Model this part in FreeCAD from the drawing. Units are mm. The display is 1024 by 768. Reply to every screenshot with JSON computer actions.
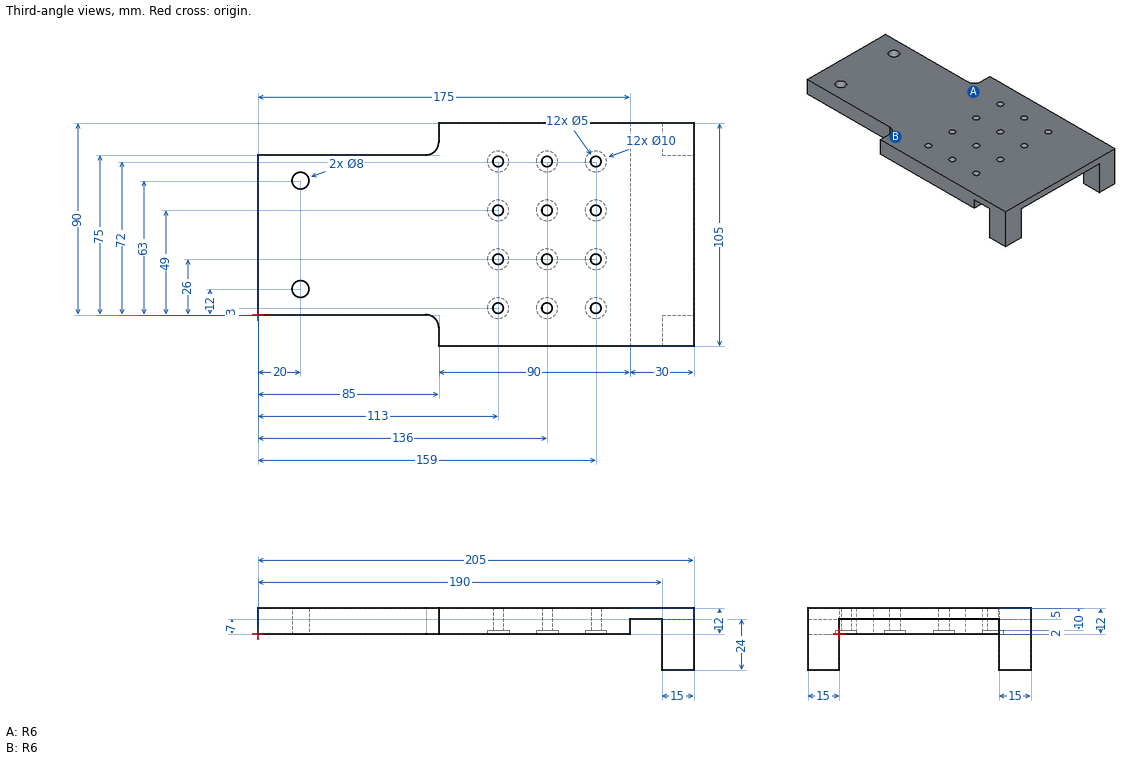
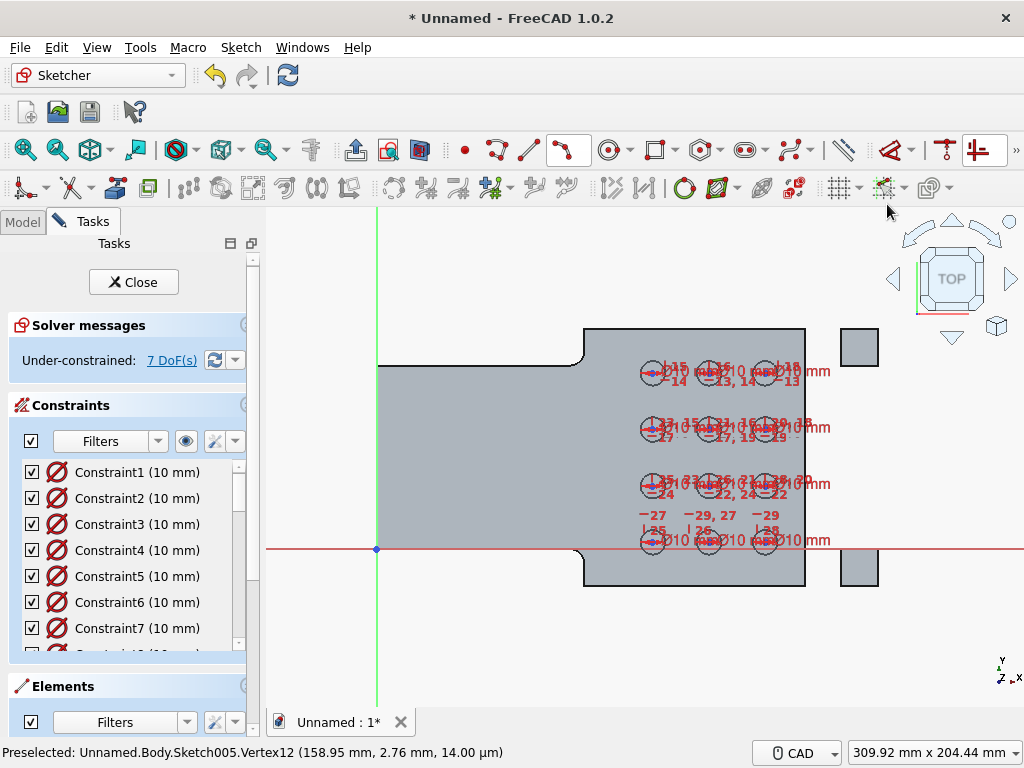
{"action": "key", "text": "d"}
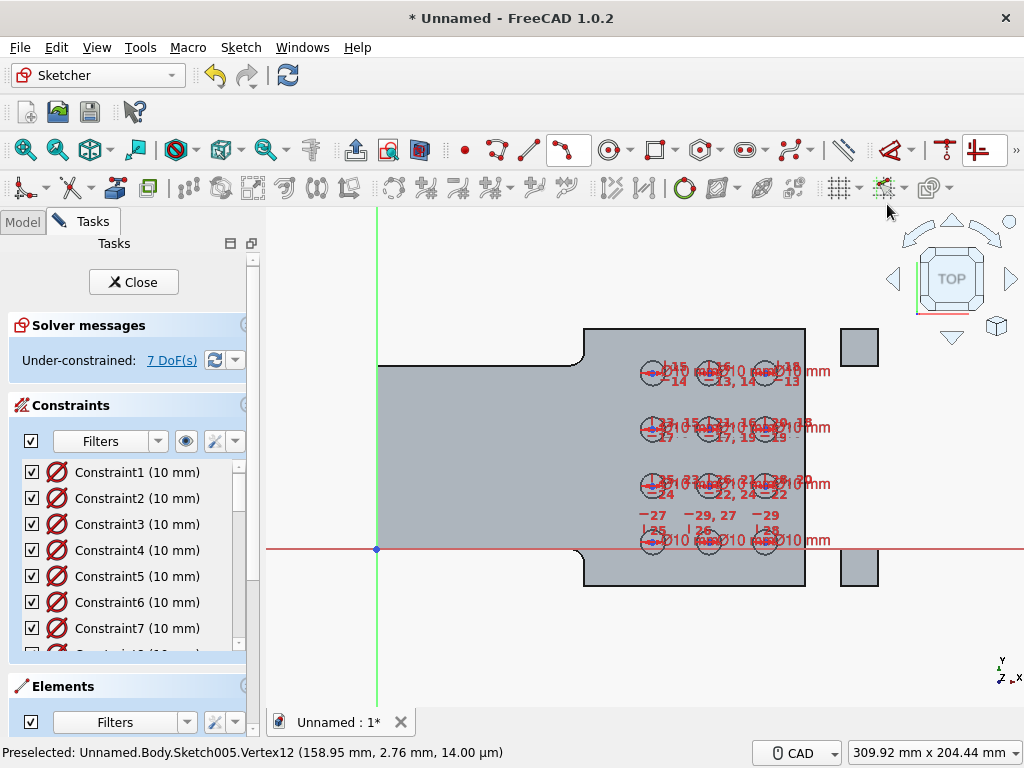
{"action": "scroll", "coordinate": [653, 542], "scroll_direction": "up", "scroll_amount": 9}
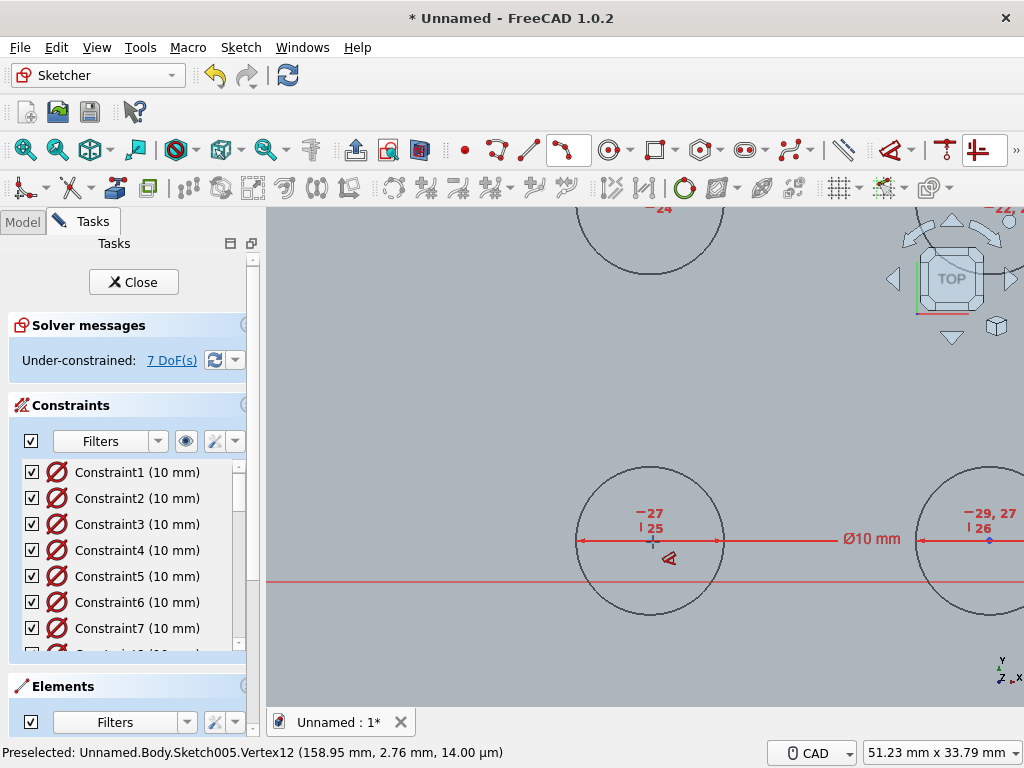
{"action": "left_click", "coordinate": [650, 541]}
{"action": "left_click", "coordinate": [684, 561]}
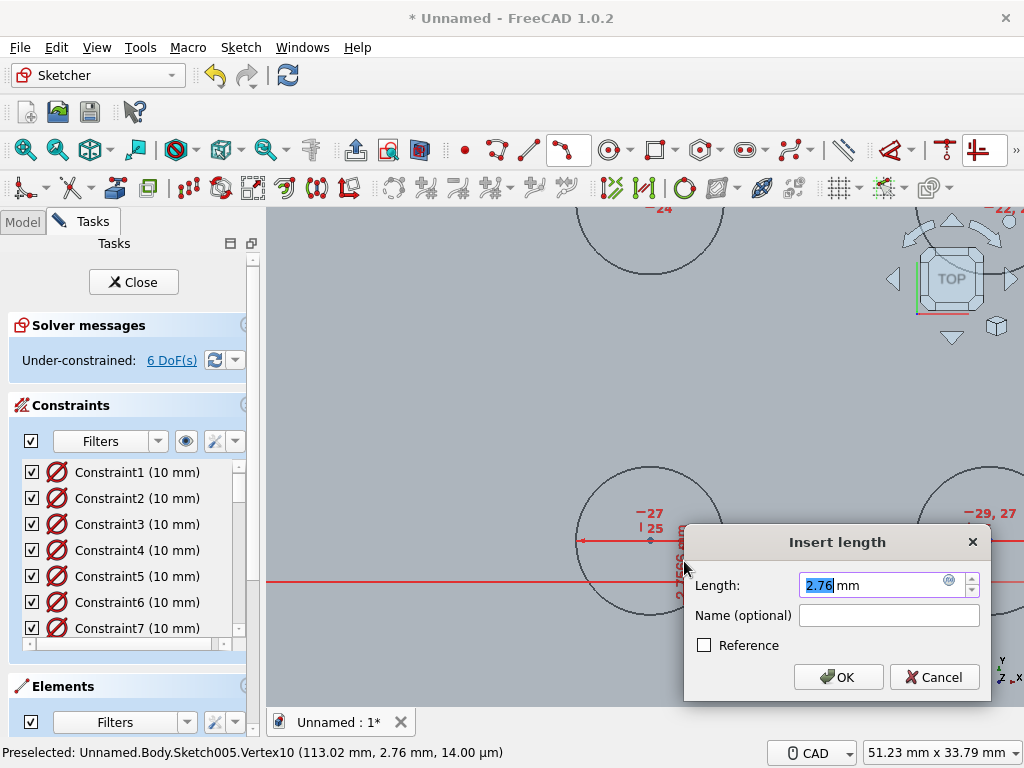
{"action": "type", "text": "3"}
{"action": "key", "text": "Return"}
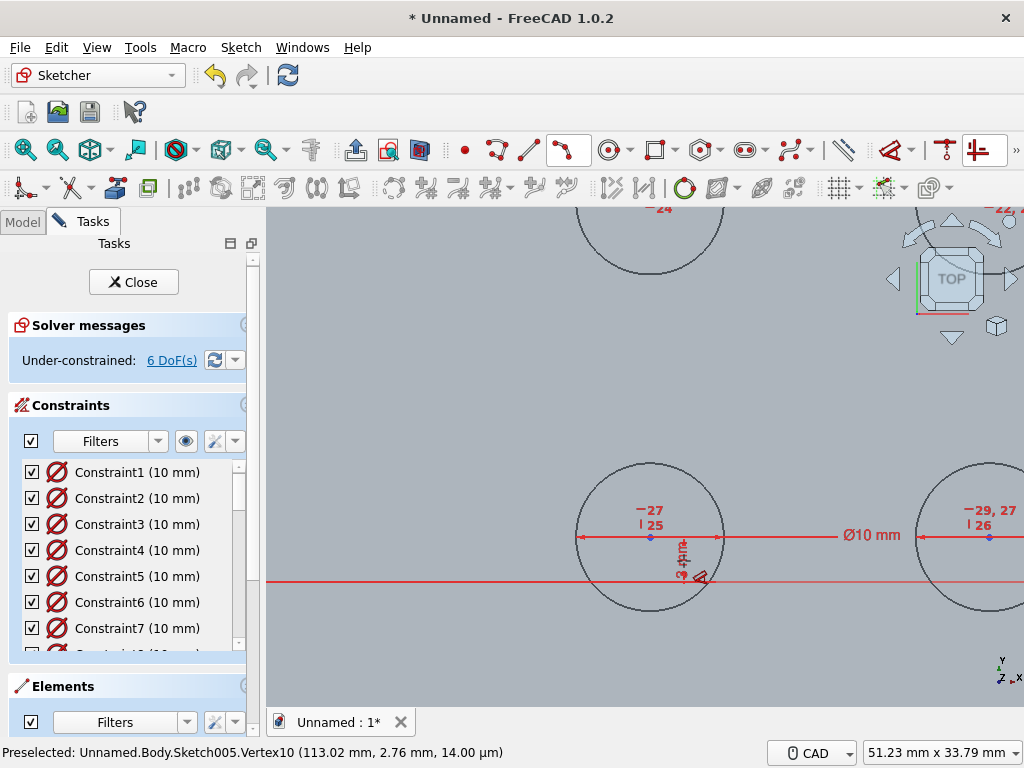
{"action": "scroll", "coordinate": [653, 542], "scroll_direction": "down", "scroll_amount": 9}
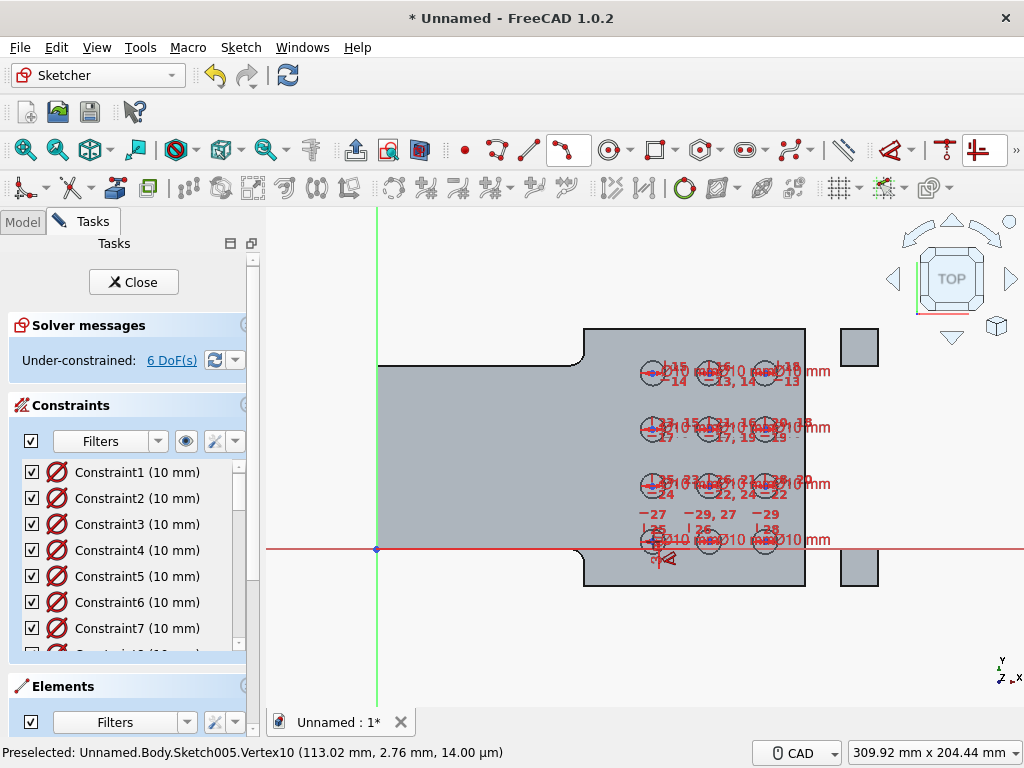
{"action": "left_click", "coordinate": [765, 373]}
{"action": "left_click", "coordinate": [343, 461]}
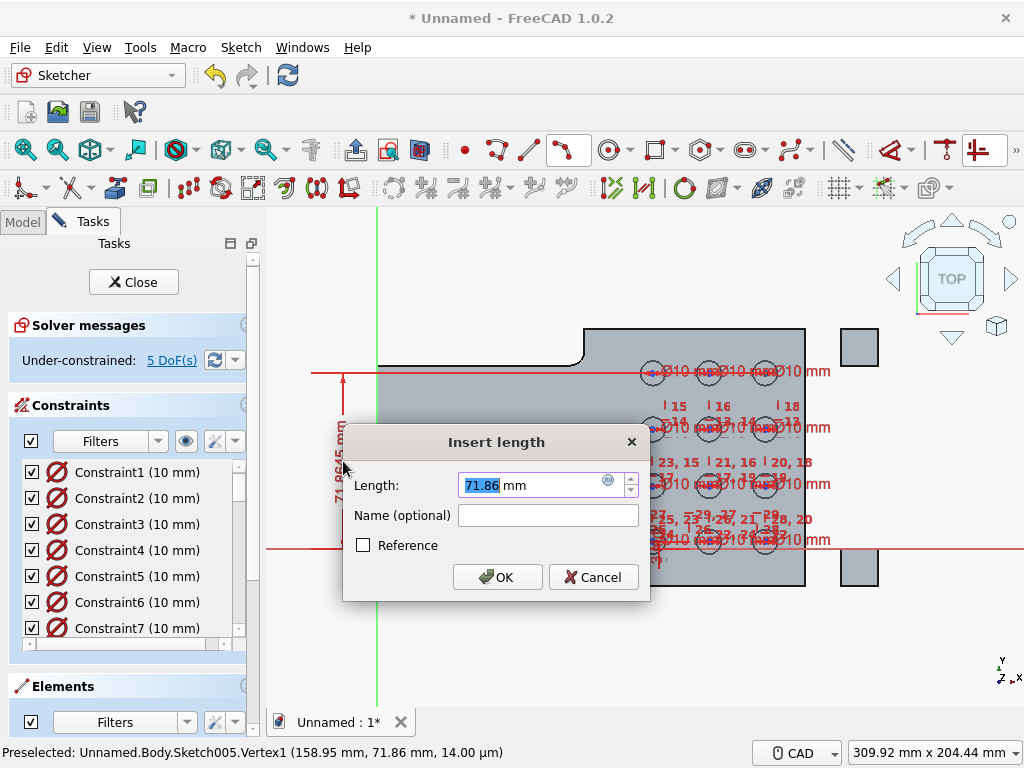
{"action": "type", "text": "72"}
{"action": "key", "text": "Return"}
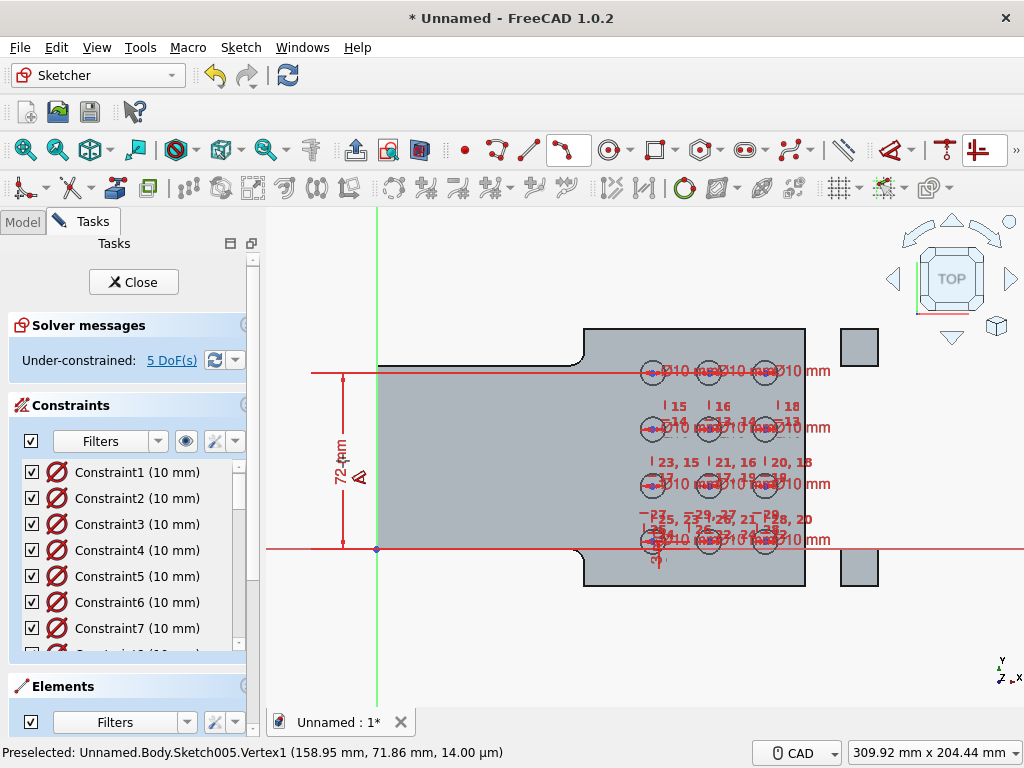
{"action": "left_click", "coordinate": [653, 430]}
{"action": "left_click", "coordinate": [343, 489]}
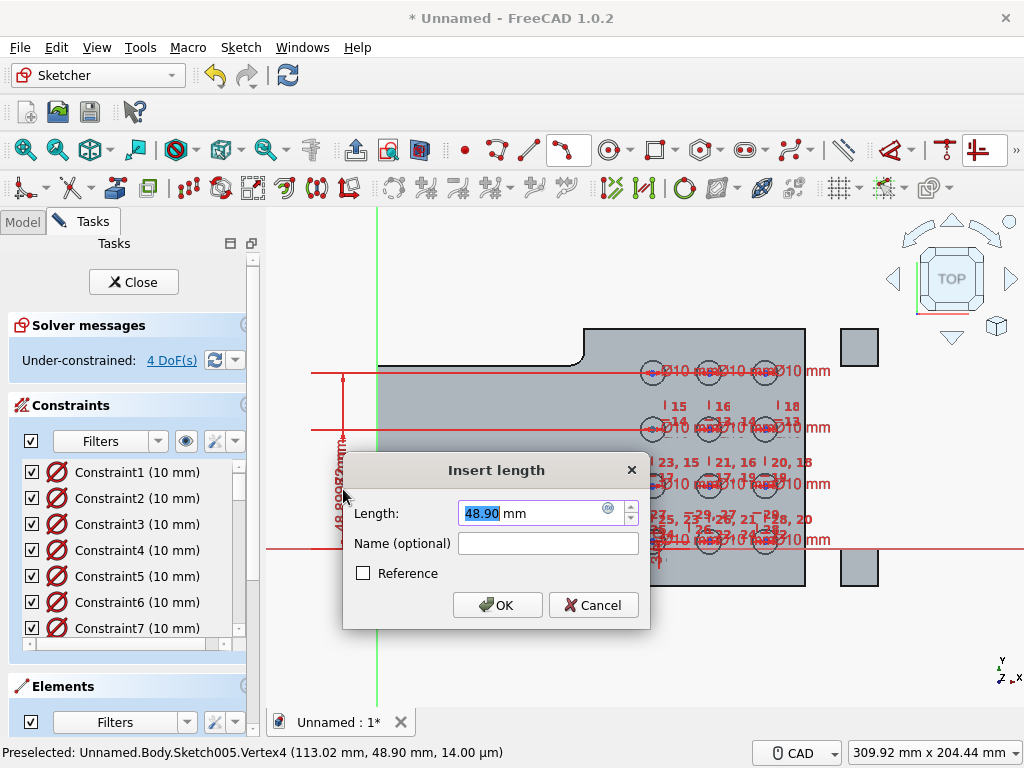
{"action": "type", "text": "49"}
{"action": "key", "text": "Return"}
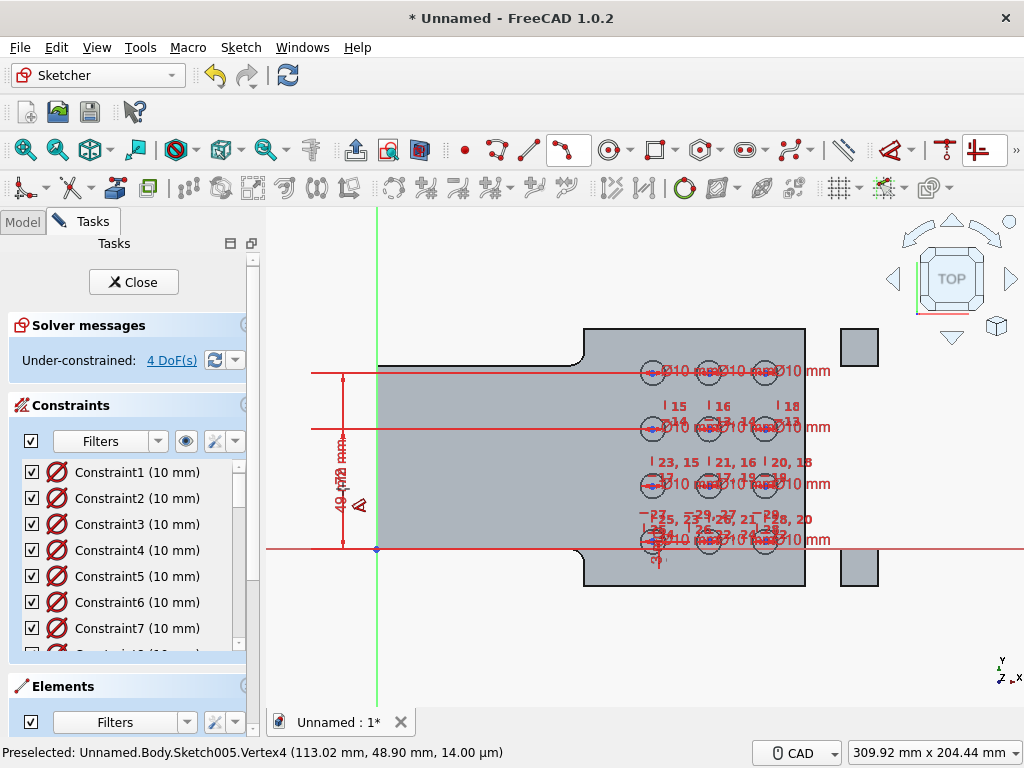
{"action": "left_click", "coordinate": [765, 486]}
{"action": "left_click", "coordinate": [343, 518]}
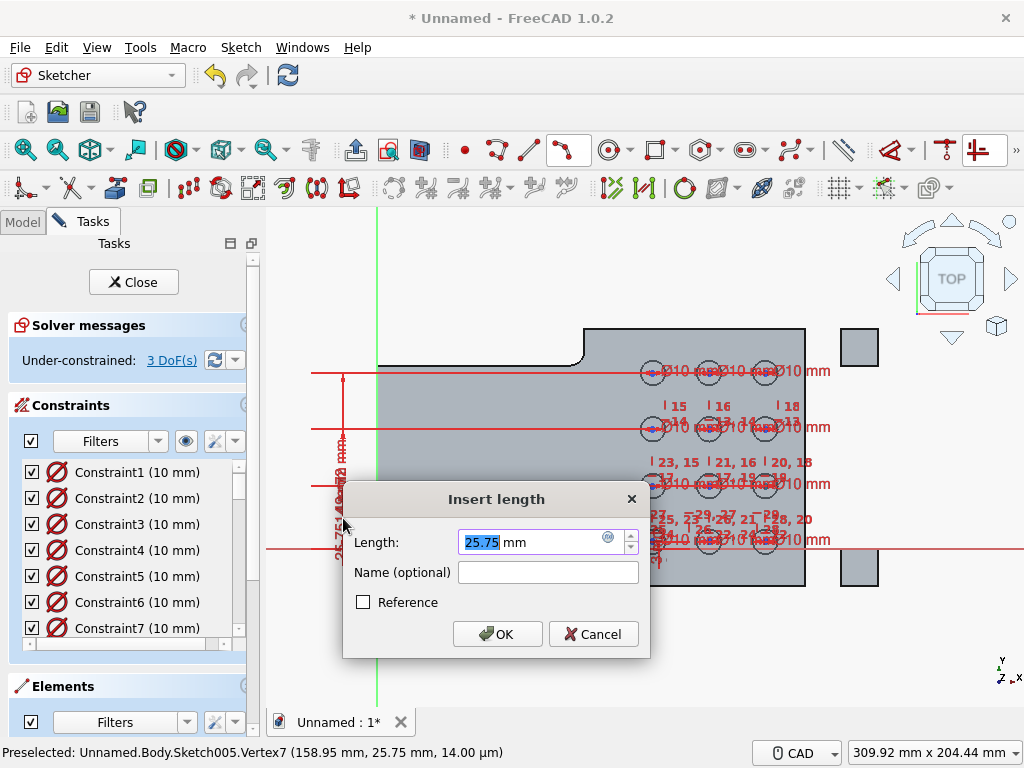
{"action": "type", "text": "26"}
{"action": "key", "text": "Return"}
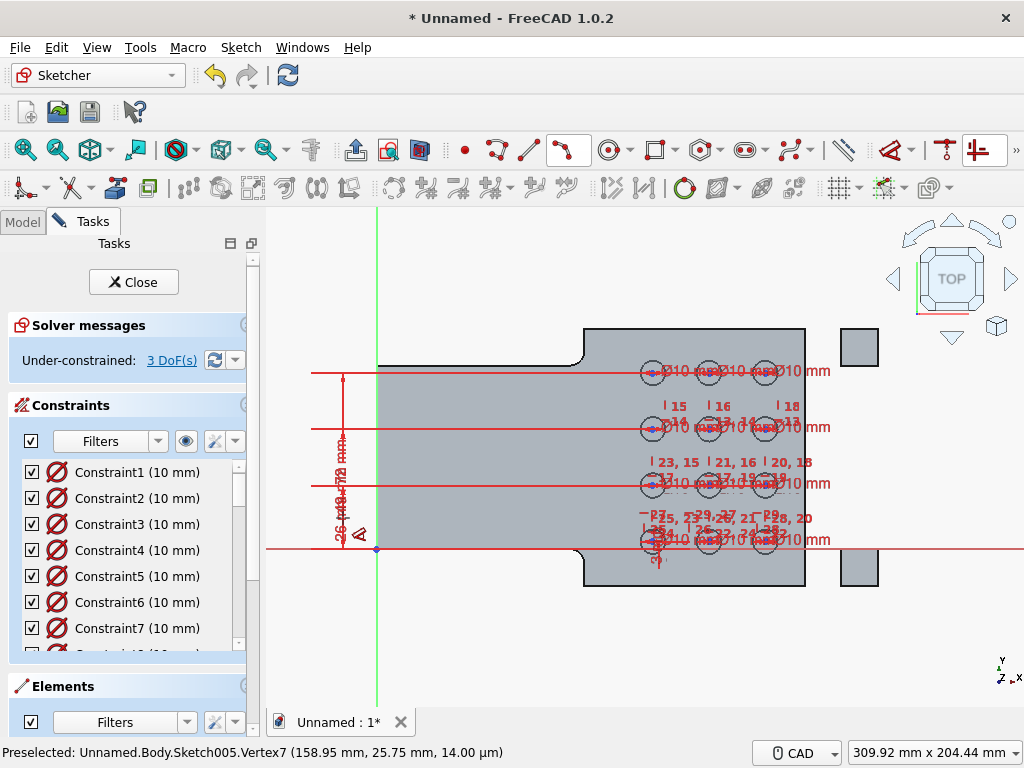
{"action": "left_click", "coordinate": [765, 373]}
{"action": "left_click", "coordinate": [571, 583]}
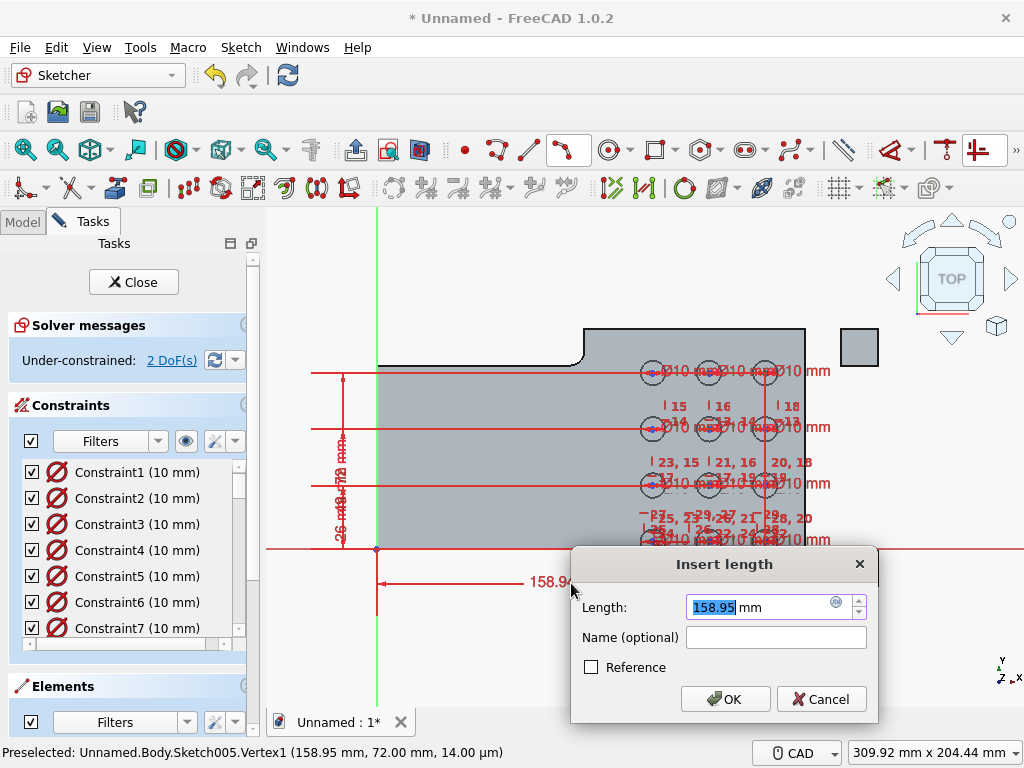
{"action": "type", "text": "159"}
{"action": "key", "text": "Return"}